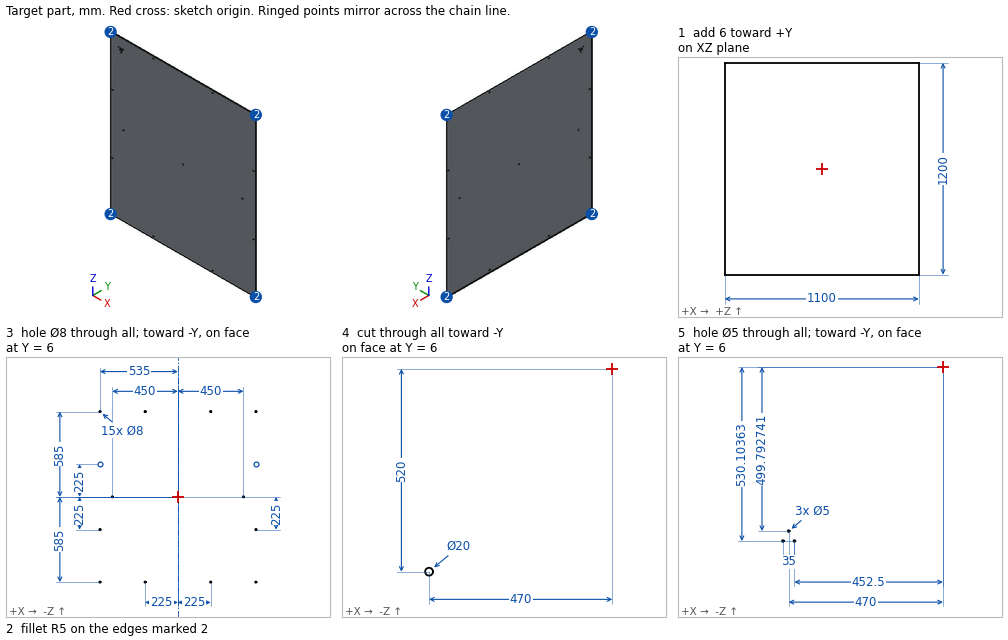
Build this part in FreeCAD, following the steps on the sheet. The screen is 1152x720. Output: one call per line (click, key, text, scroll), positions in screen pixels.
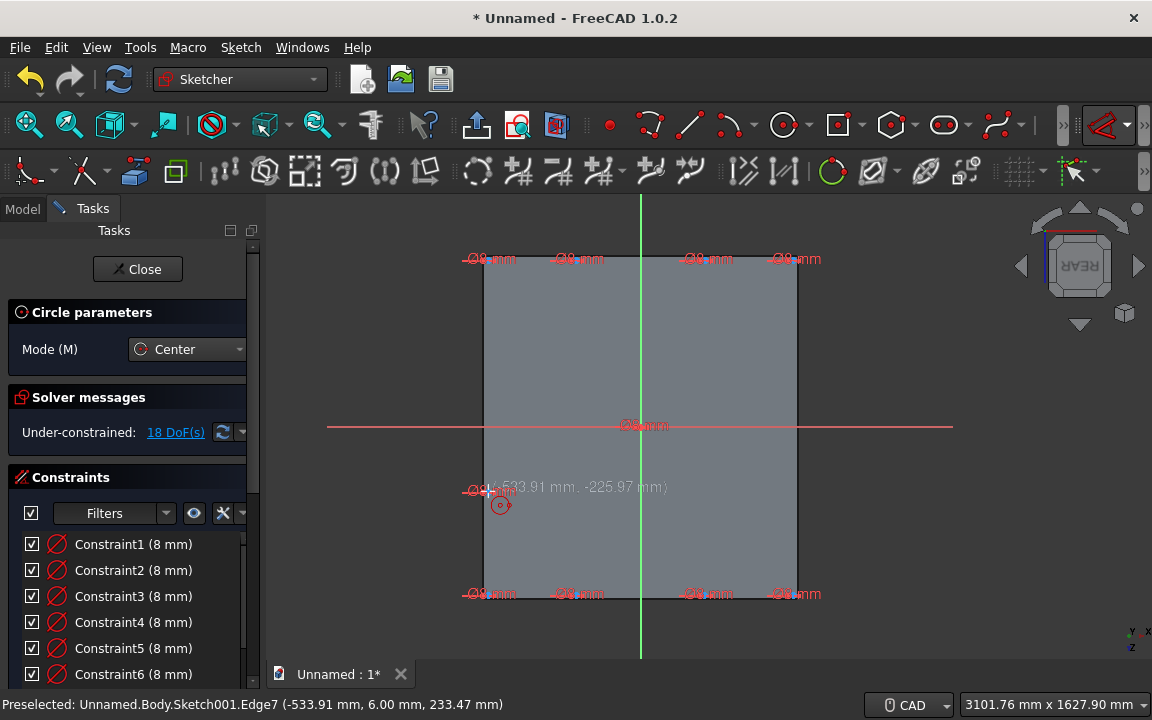
scroll(488, 363, up, 15)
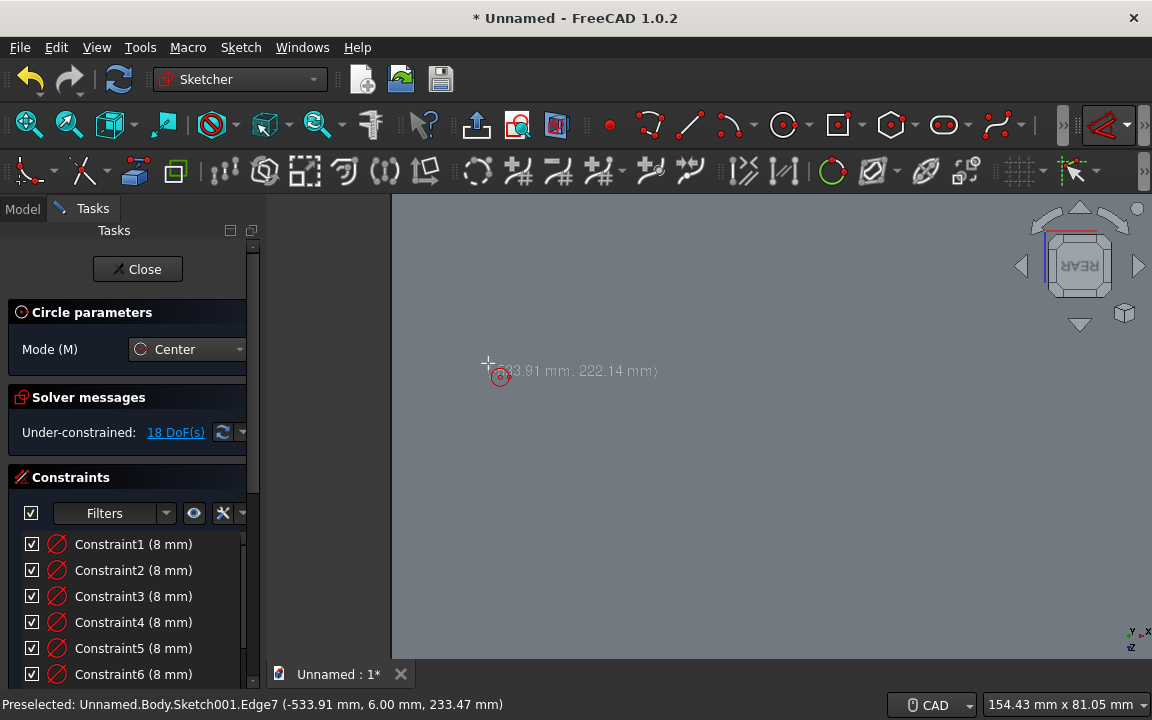
scroll(488, 362, down, 15)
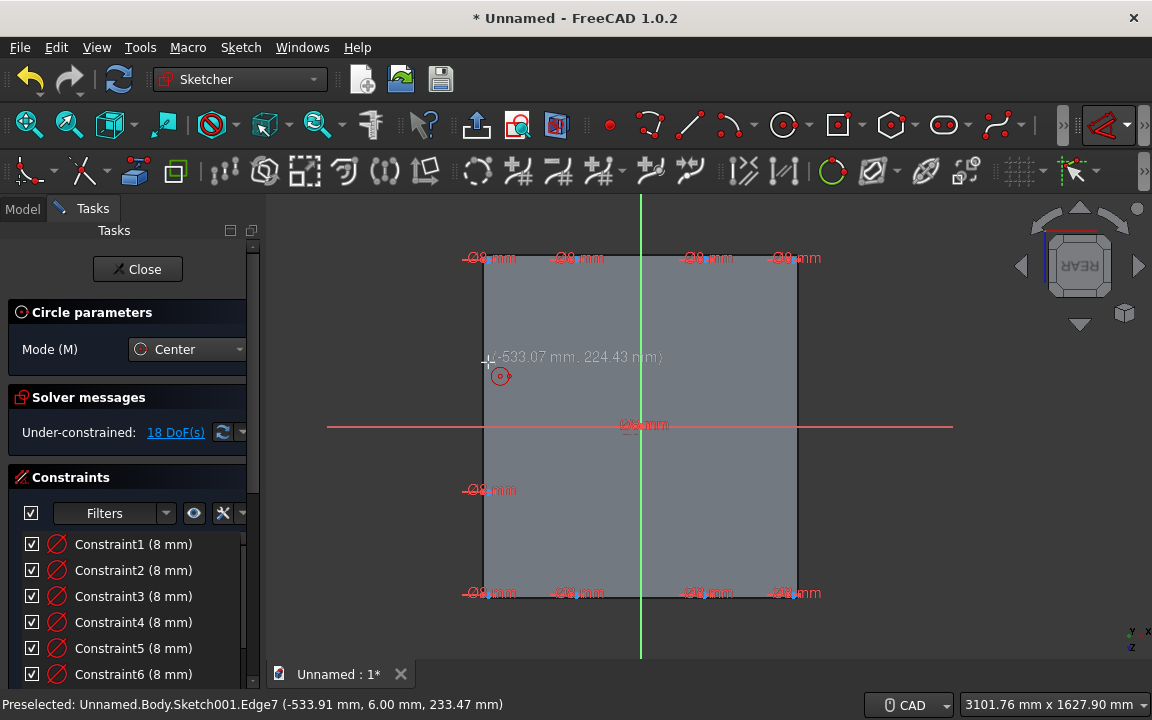
click(488, 362)
move(488, 361)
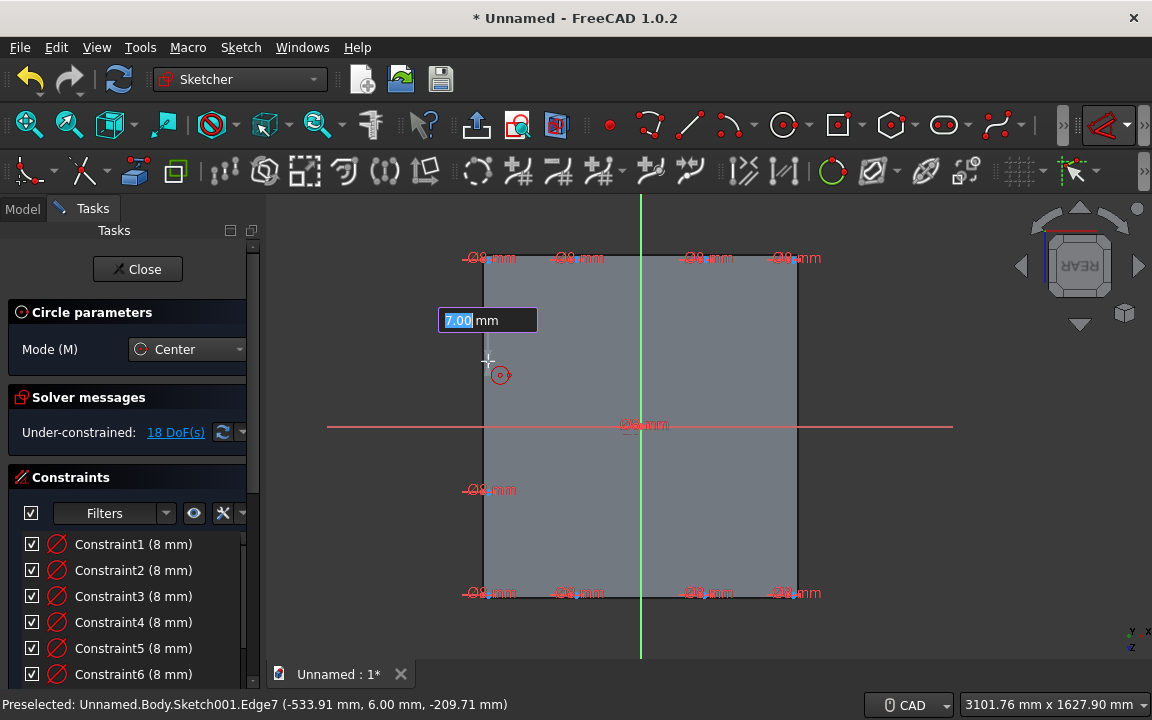
text(8)
key(Return)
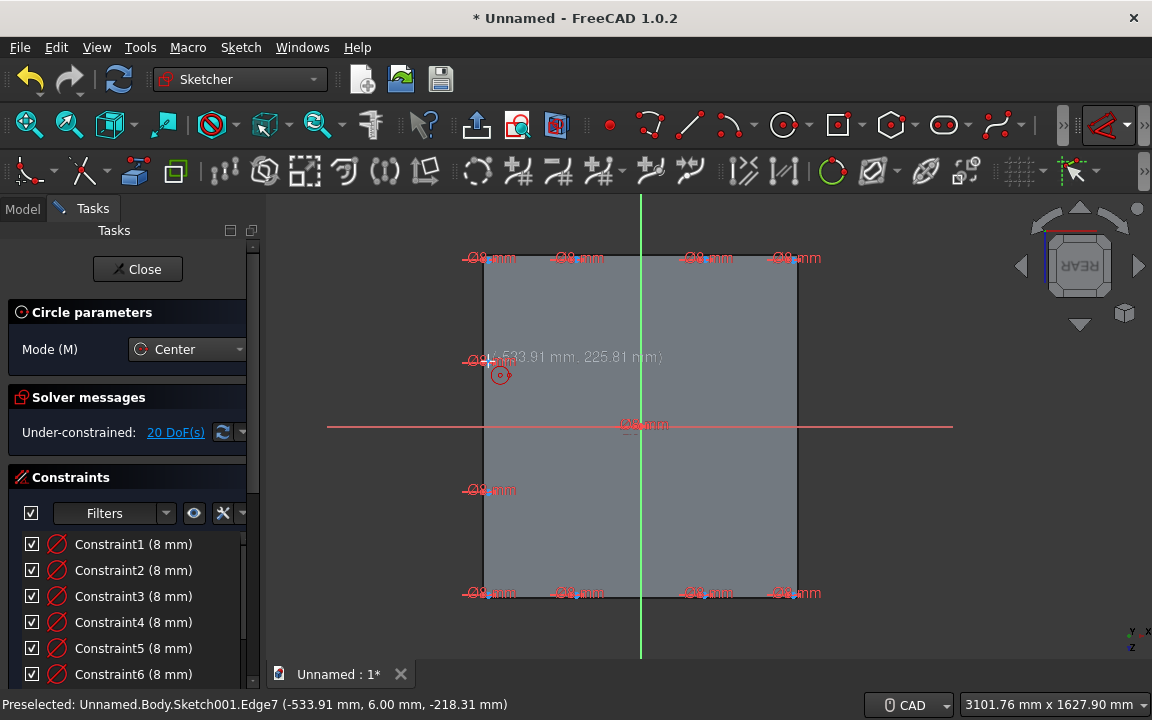
scroll(793, 362, up, 15)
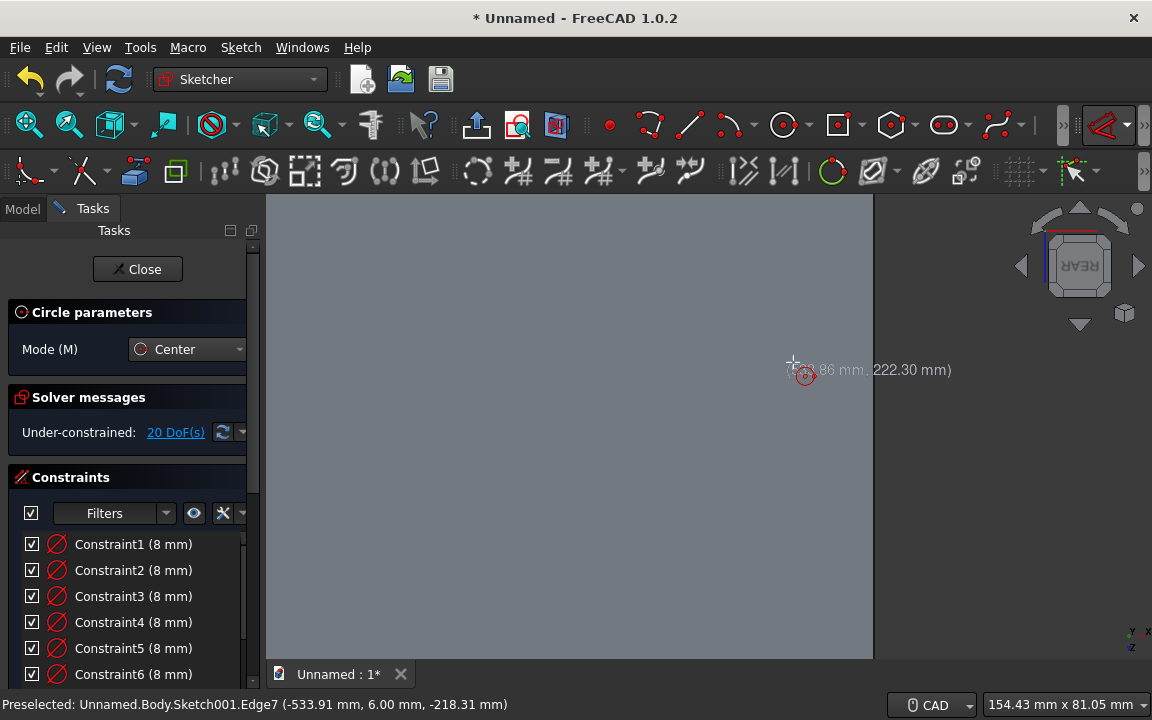
scroll(794, 362, down, 15)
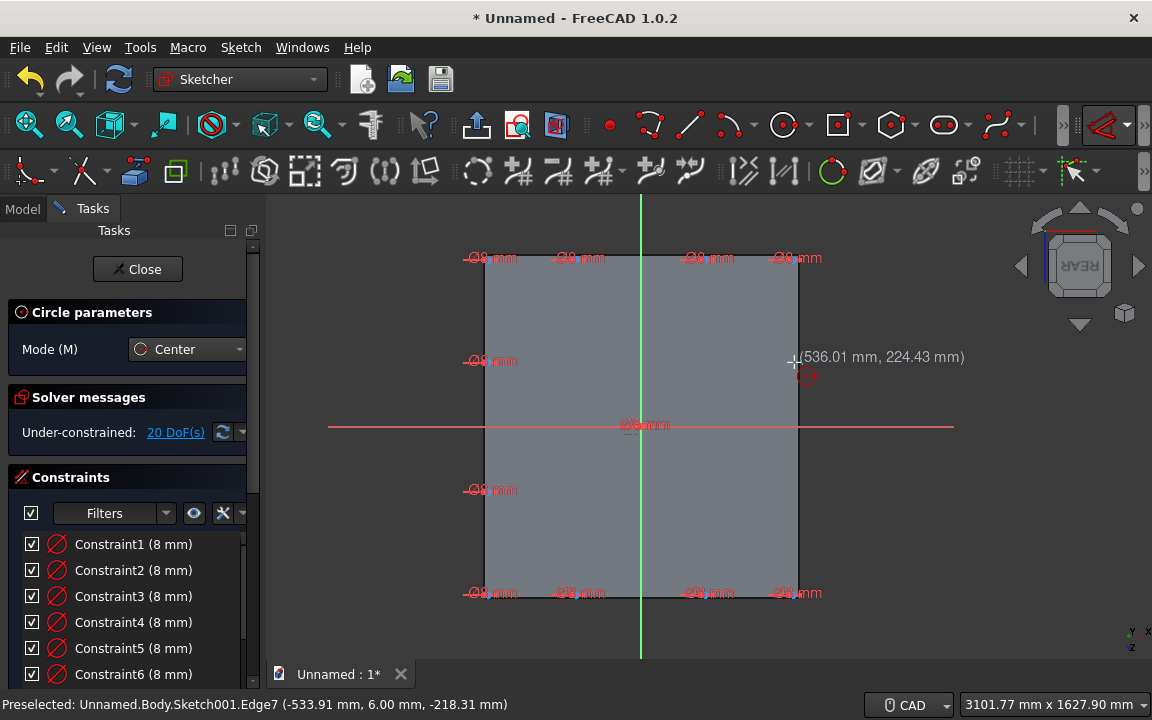
click(794, 362)
move(795, 361)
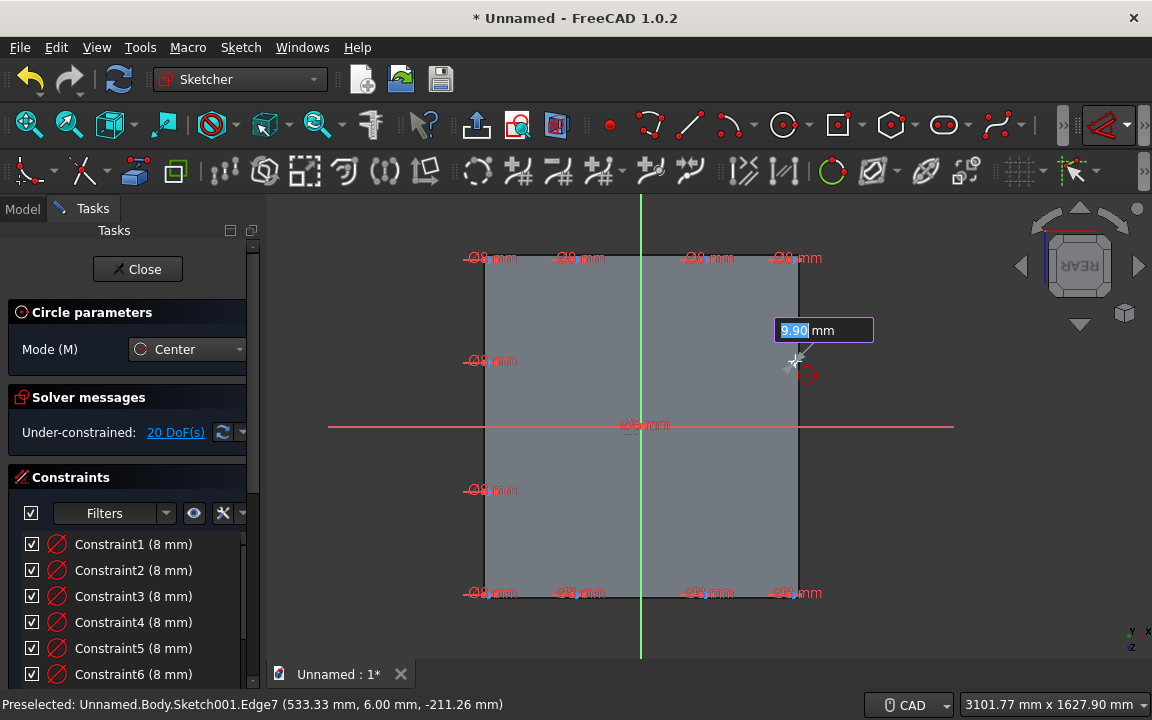
text(8)
key(Return)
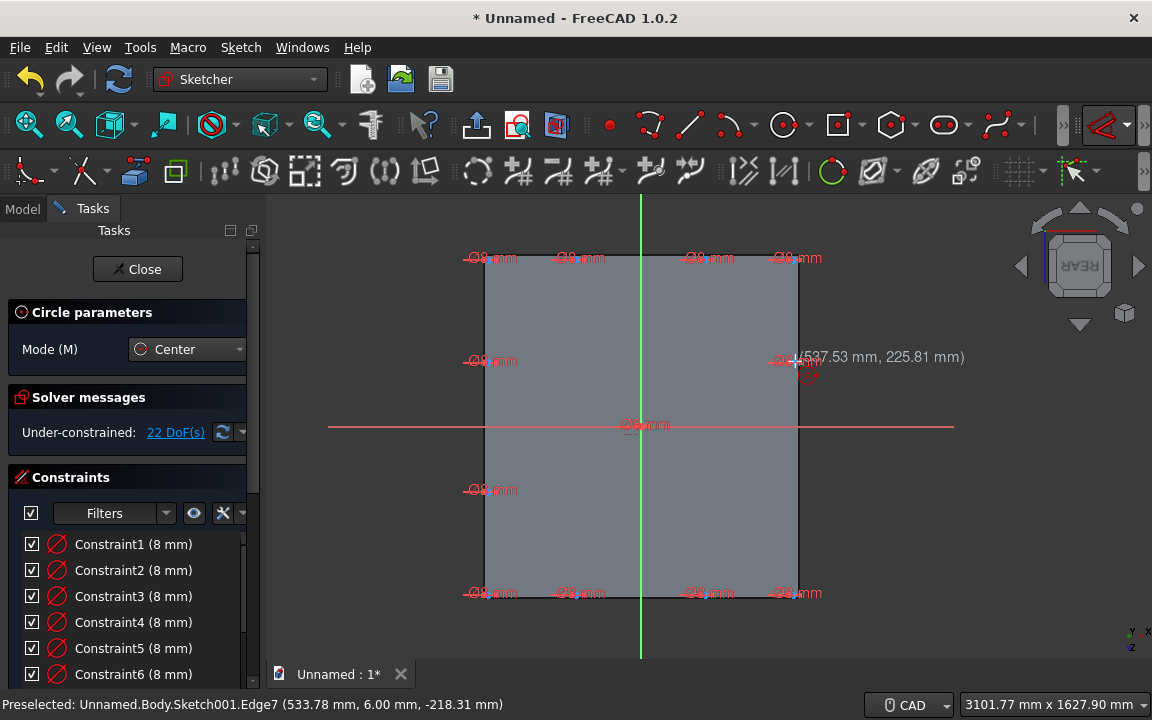
scroll(794, 491, up, 15)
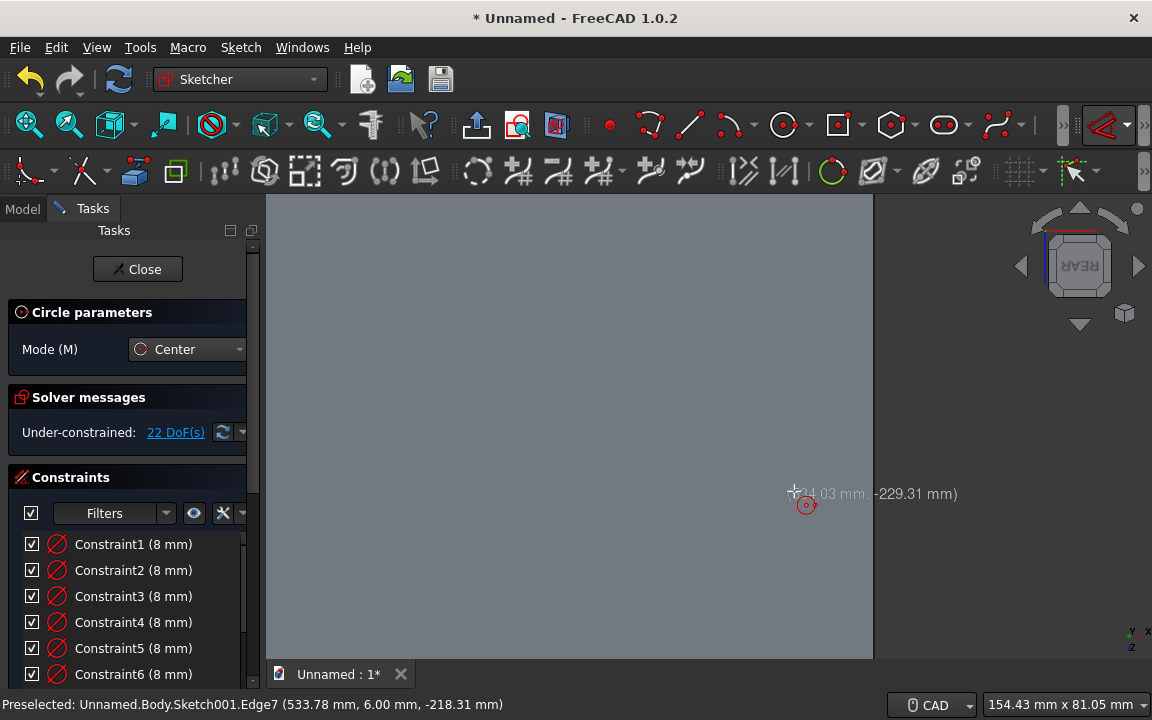
scroll(794, 492, down, 15)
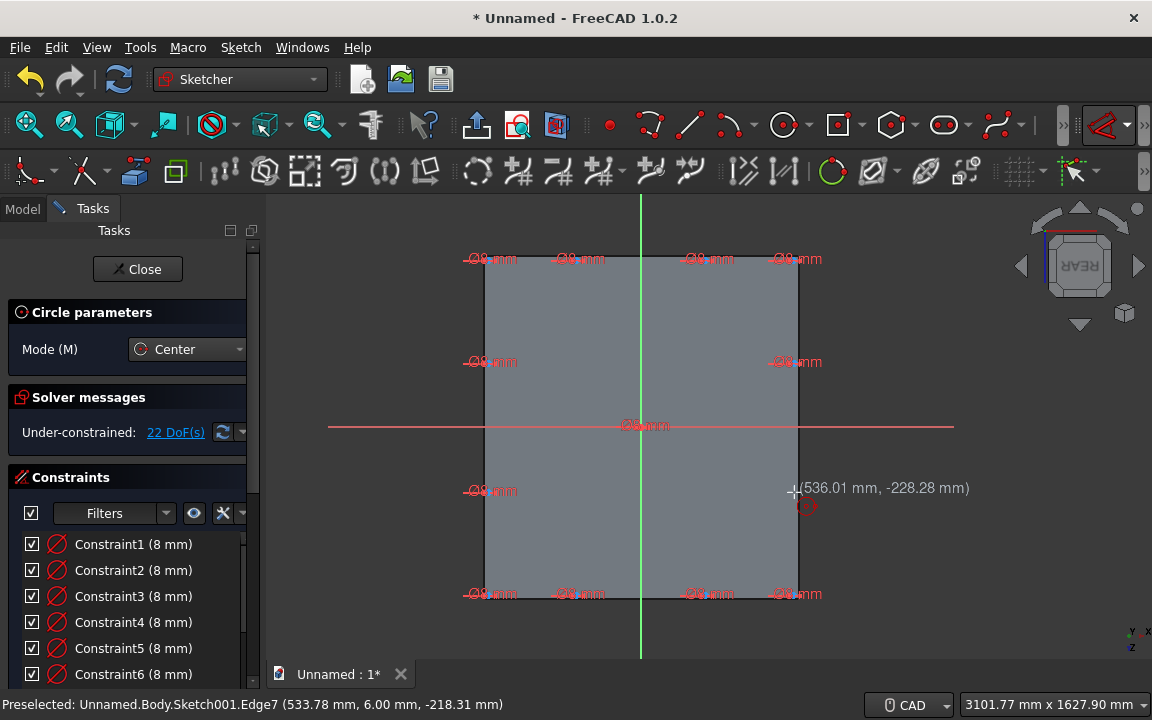
click(794, 492)
move(795, 491)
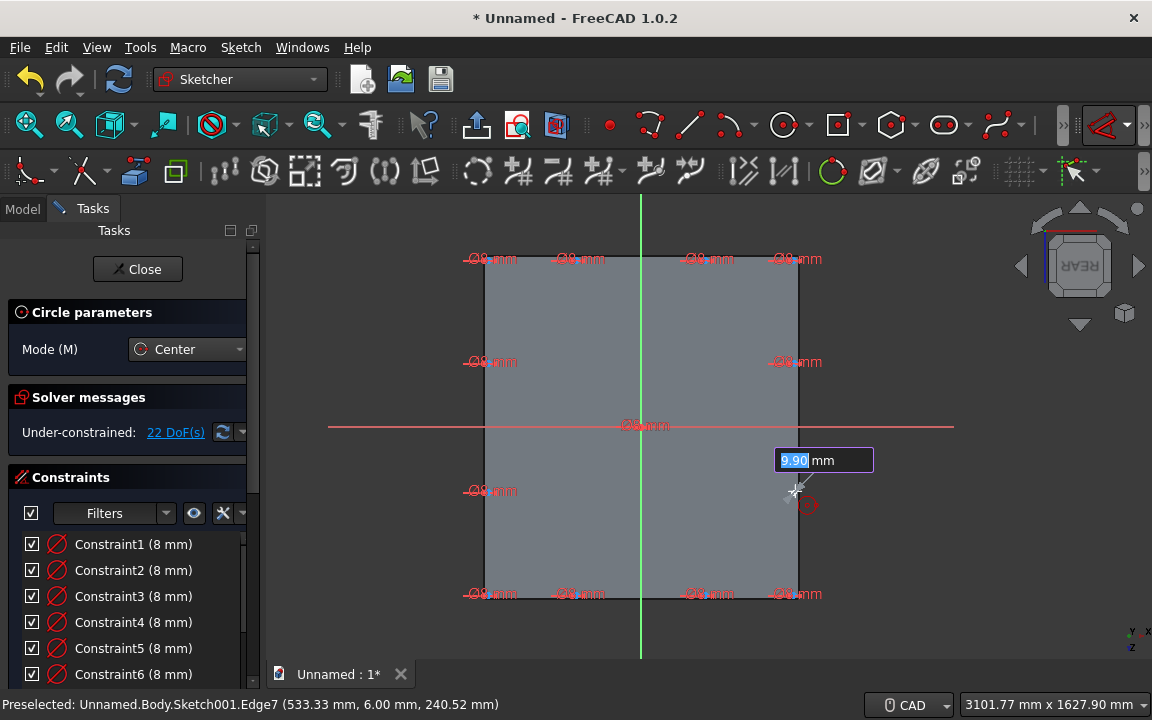
text(8)
key(Return)